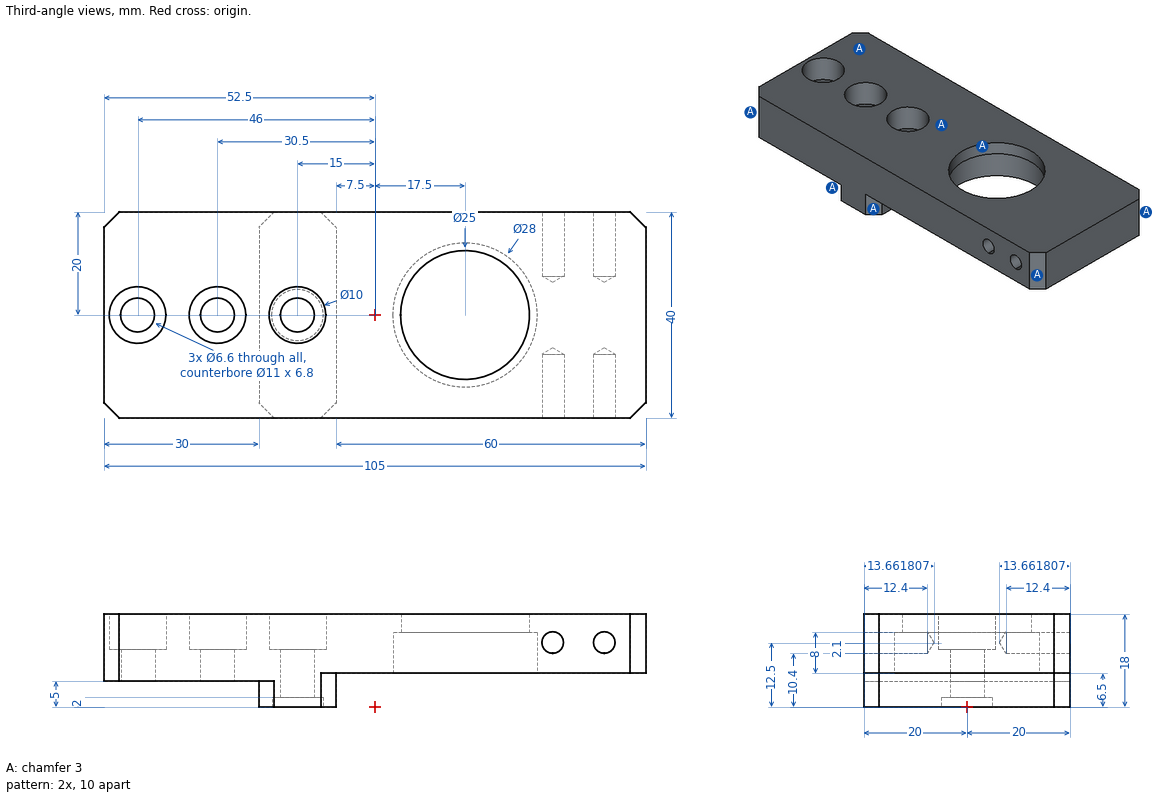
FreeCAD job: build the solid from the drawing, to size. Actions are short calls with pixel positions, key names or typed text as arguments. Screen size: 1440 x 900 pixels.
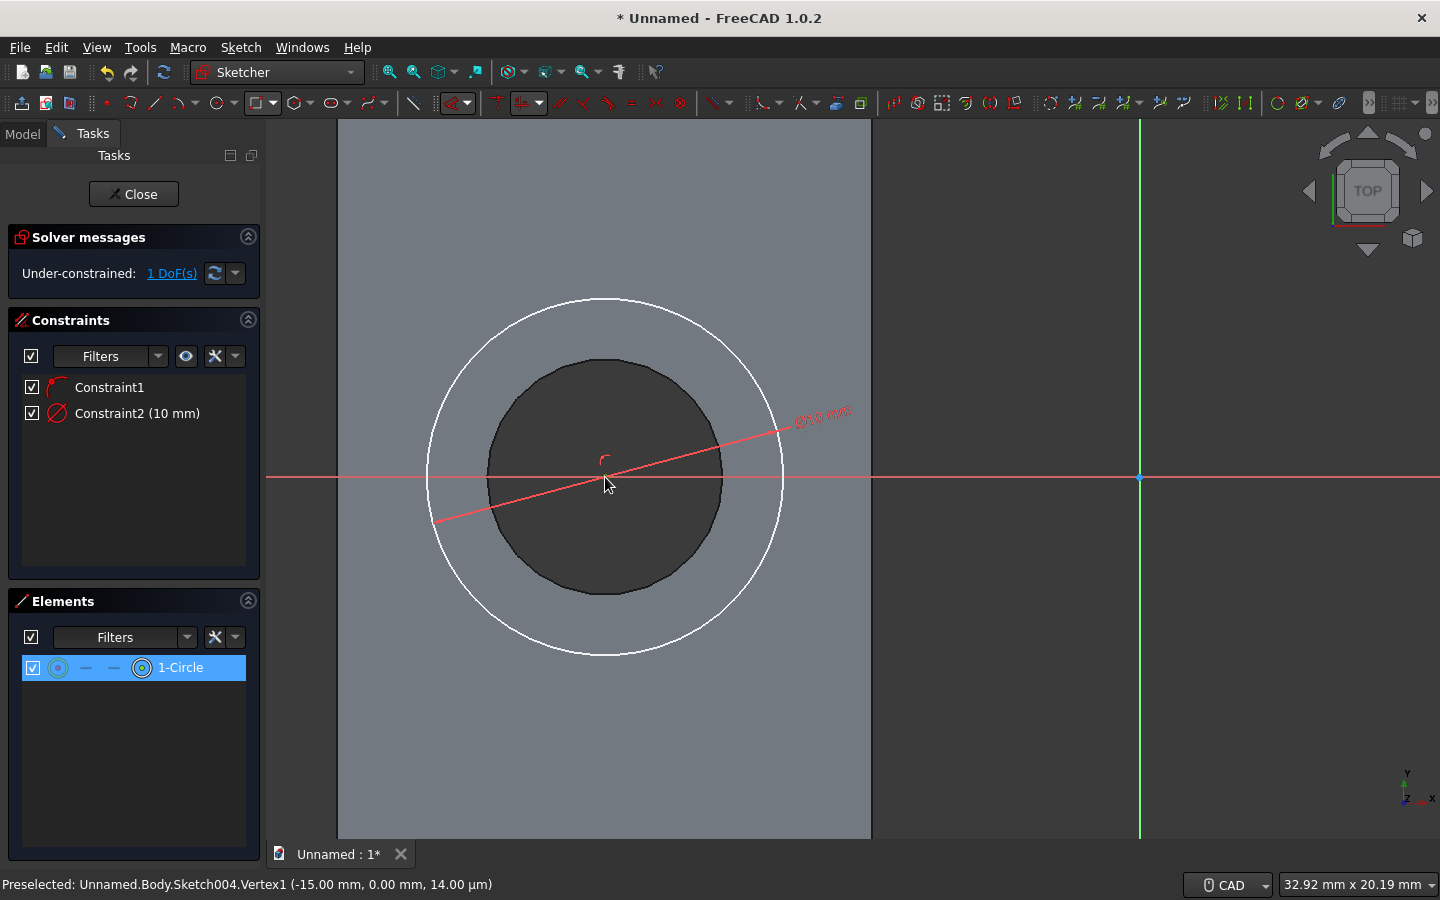
click(470, 104)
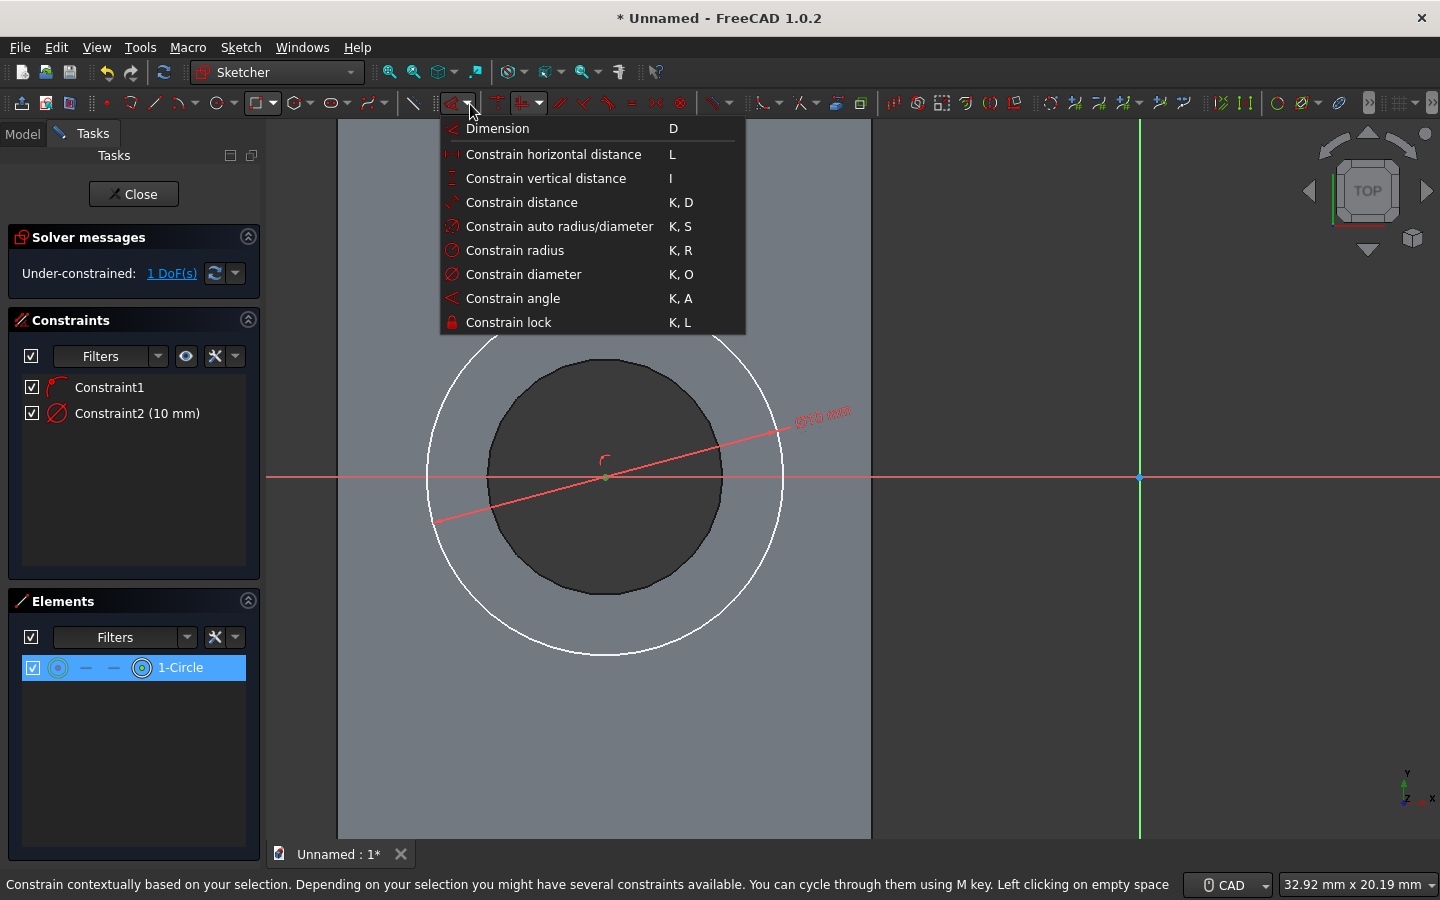
click(593, 154)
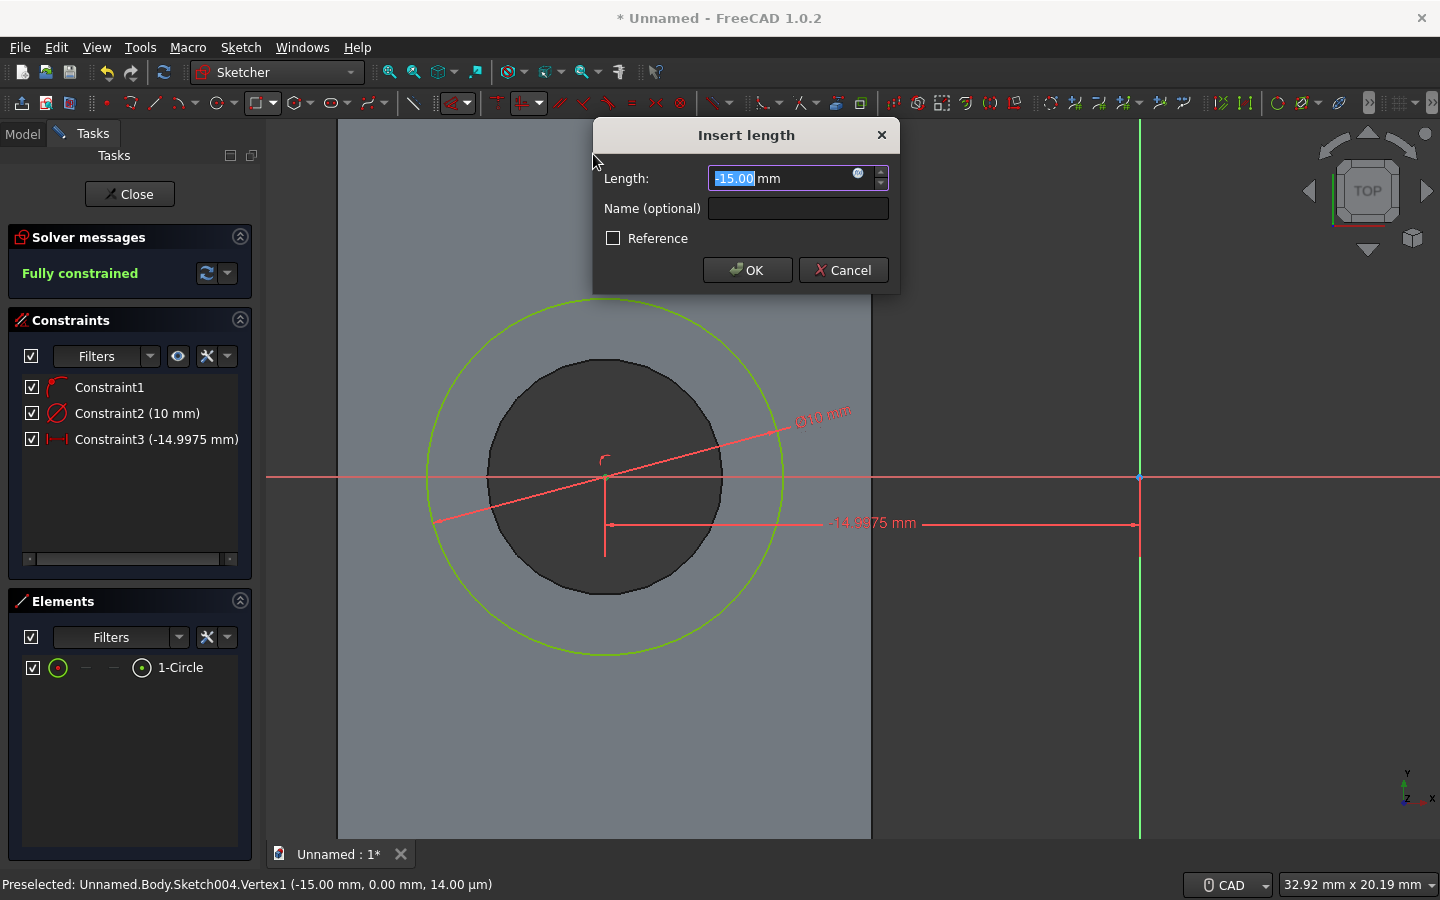
text(-15)
key(Return)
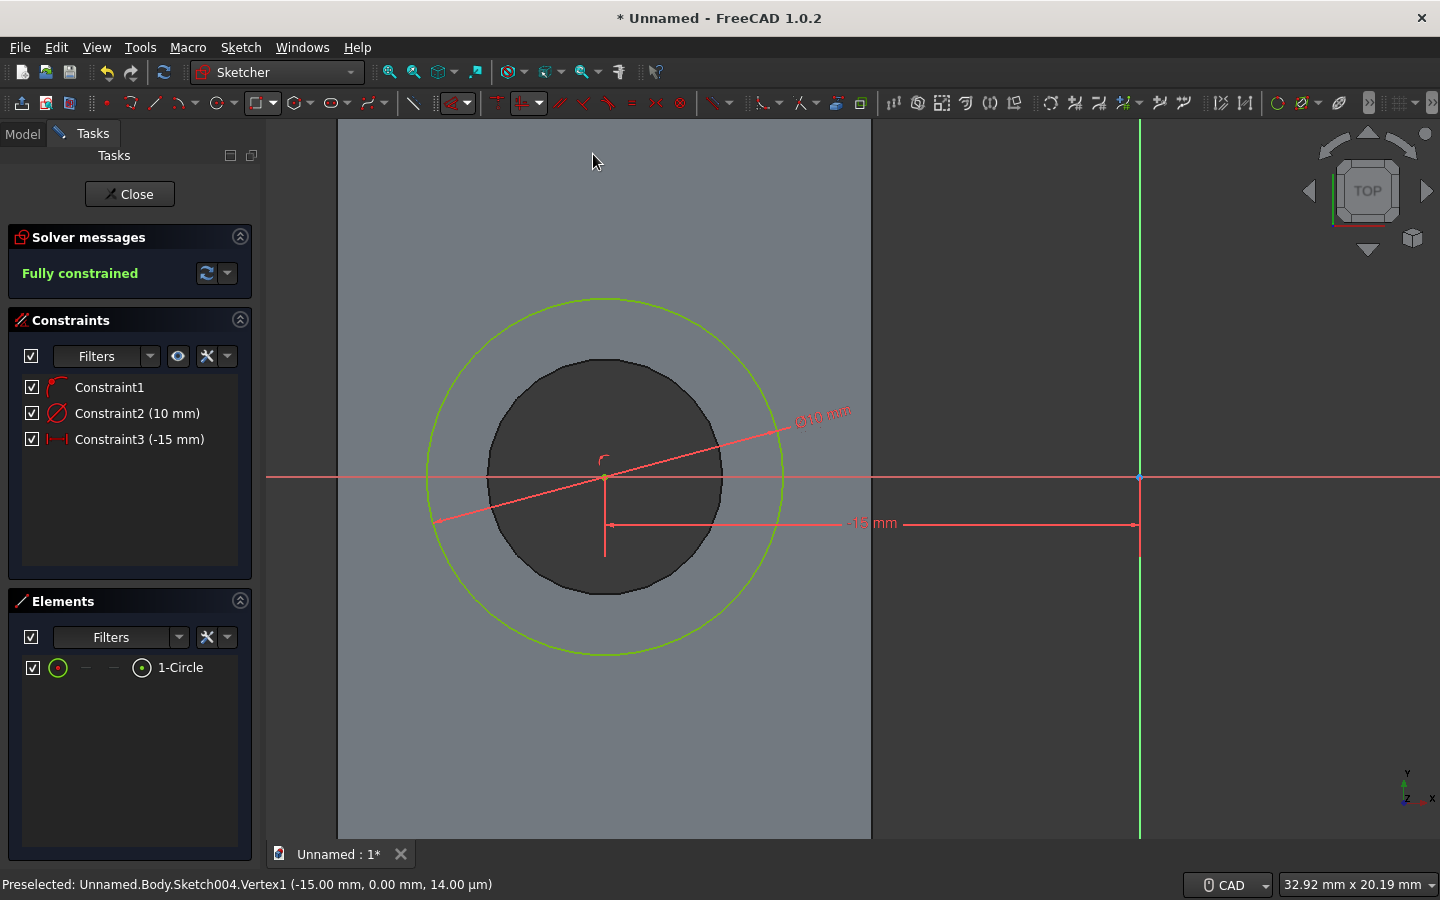
click(130, 194)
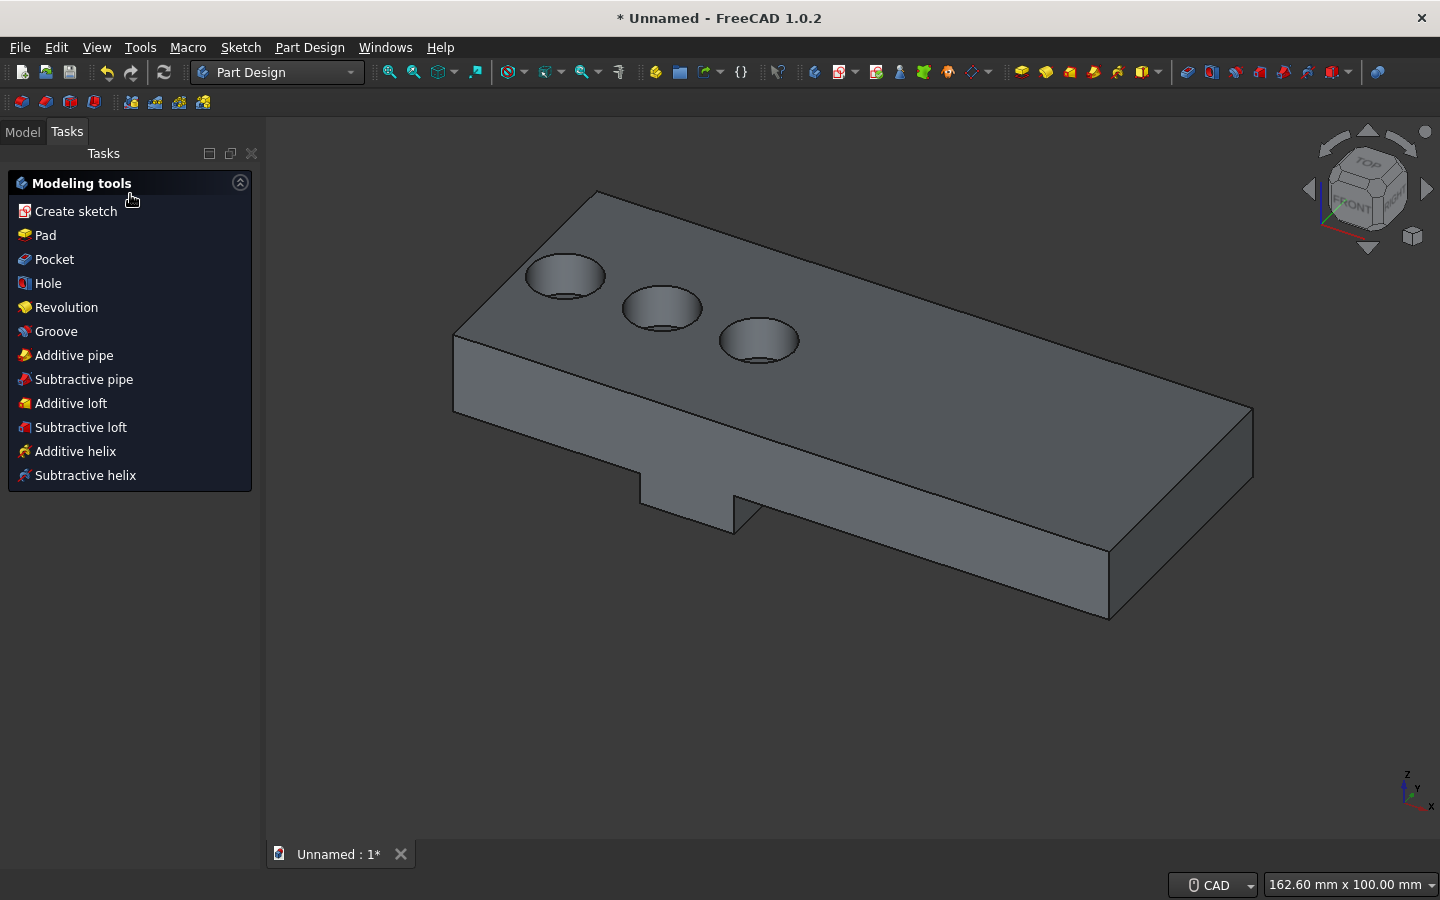
click(1188, 72)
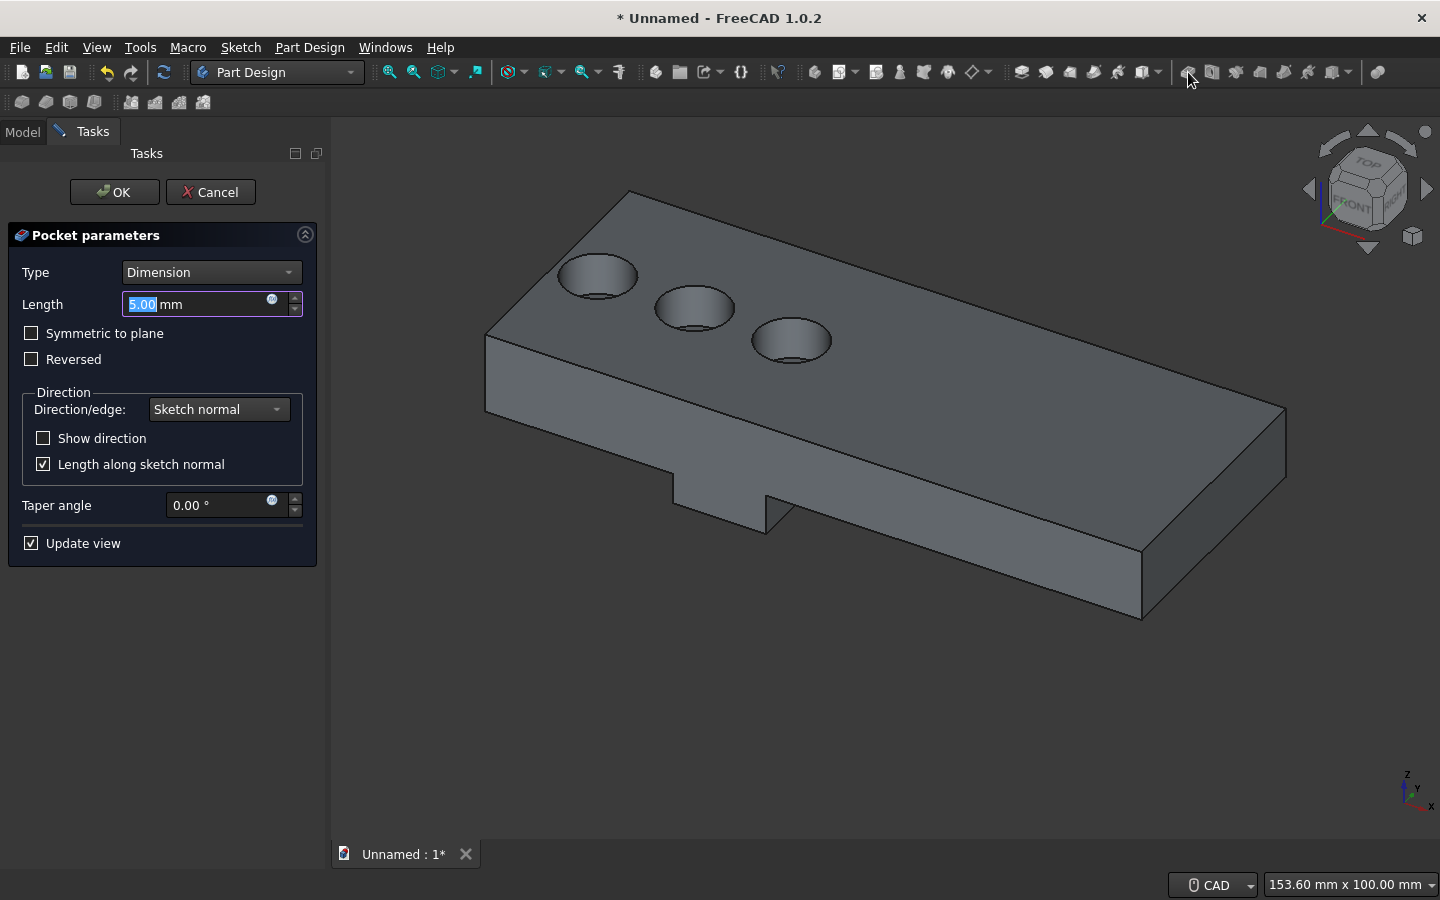
text(2)
key(Tab)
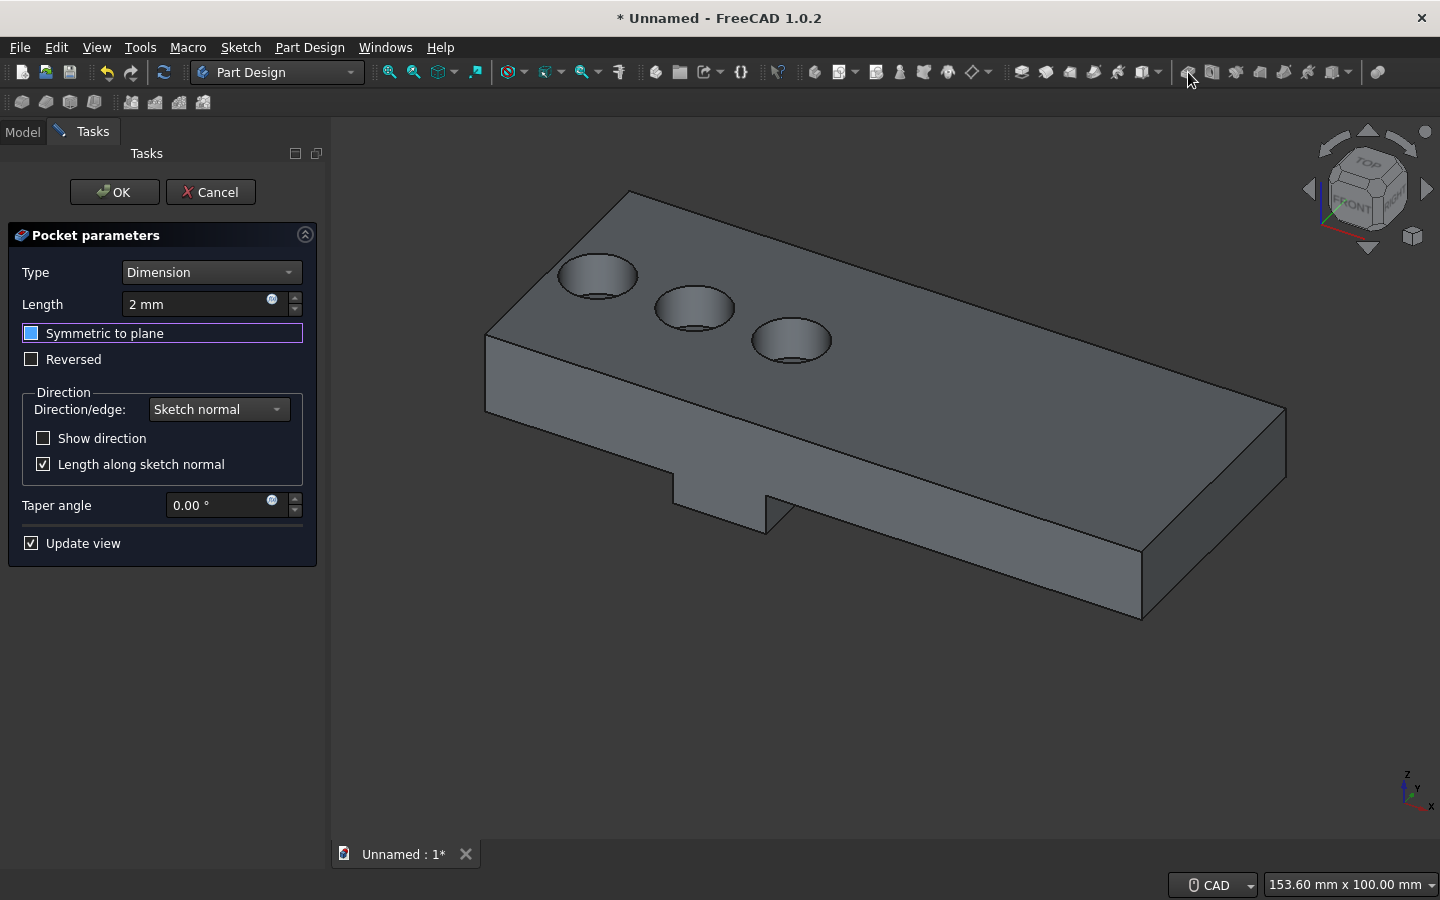
click(30, 359)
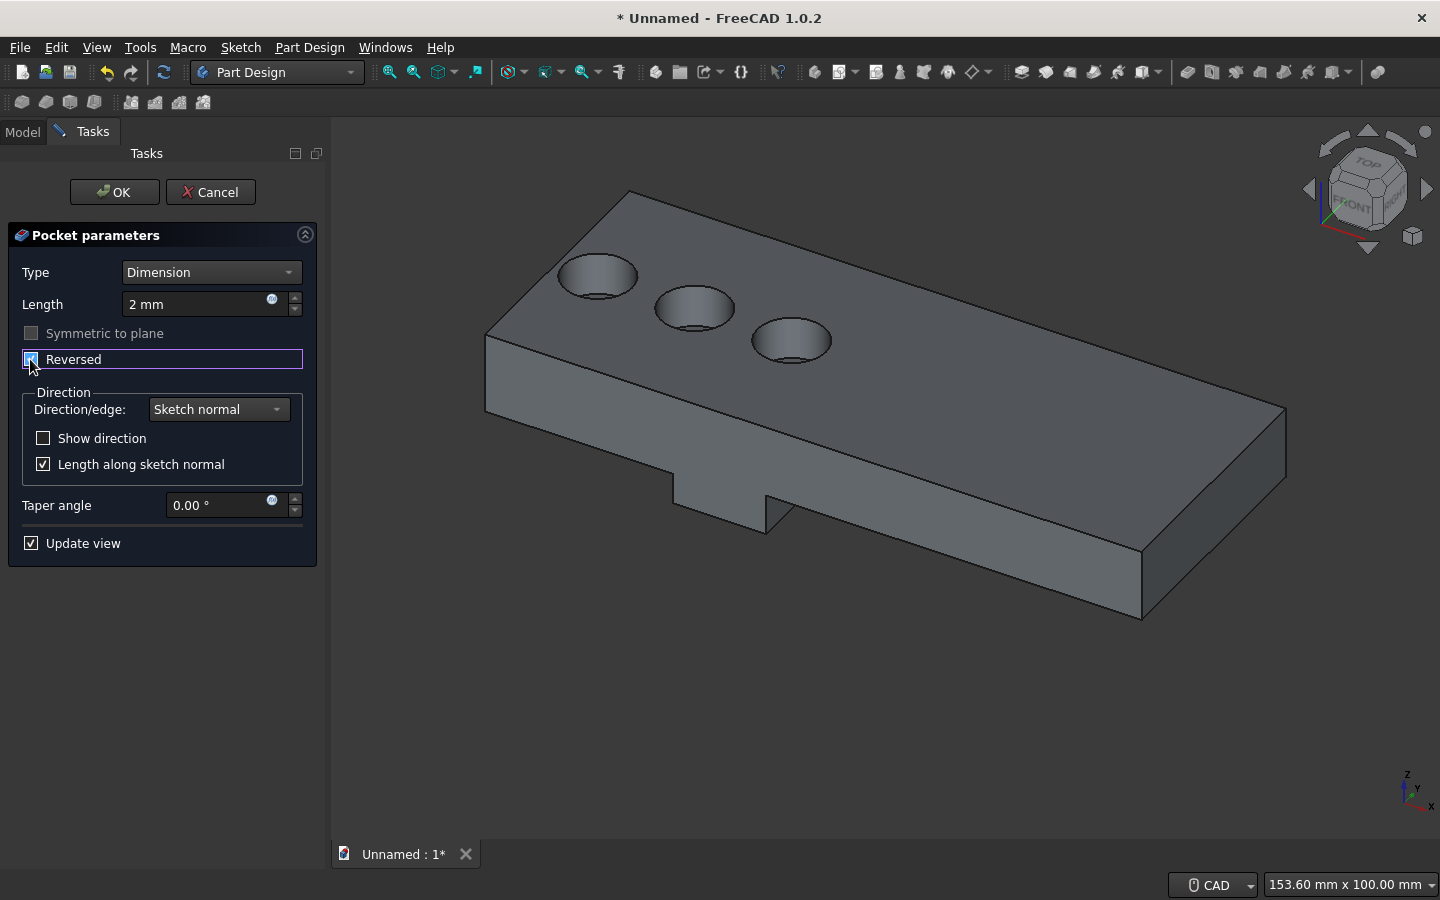
click(115, 192)